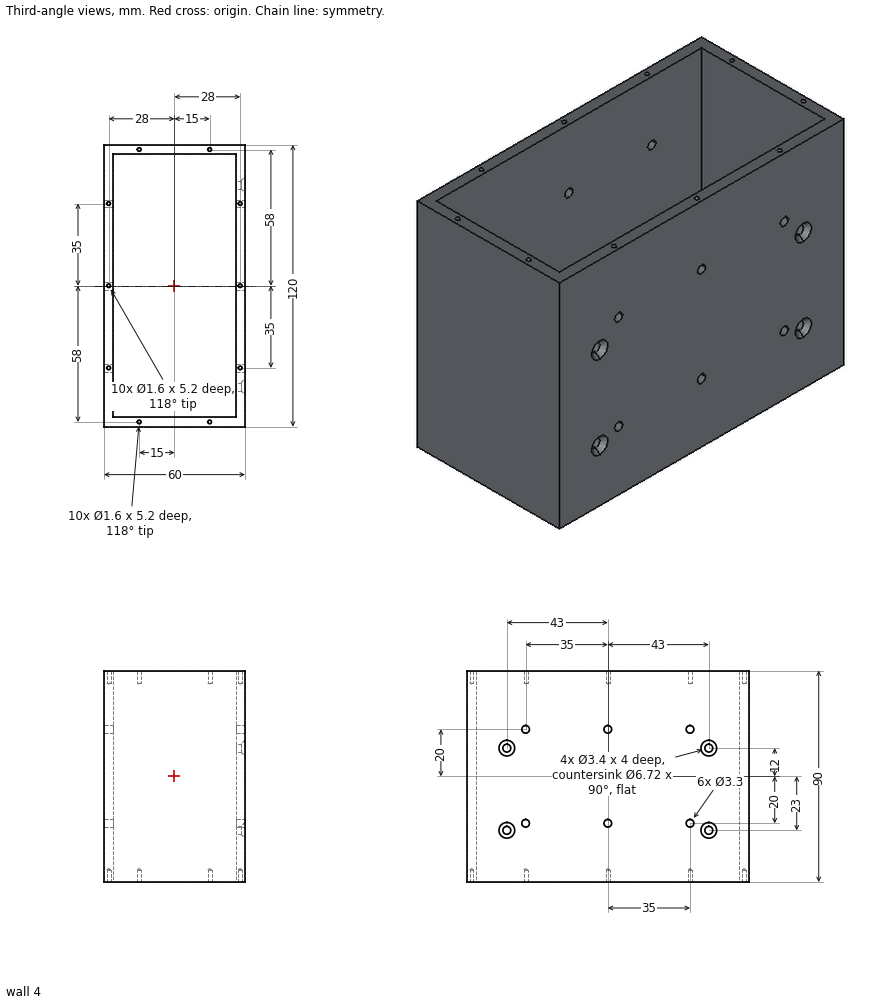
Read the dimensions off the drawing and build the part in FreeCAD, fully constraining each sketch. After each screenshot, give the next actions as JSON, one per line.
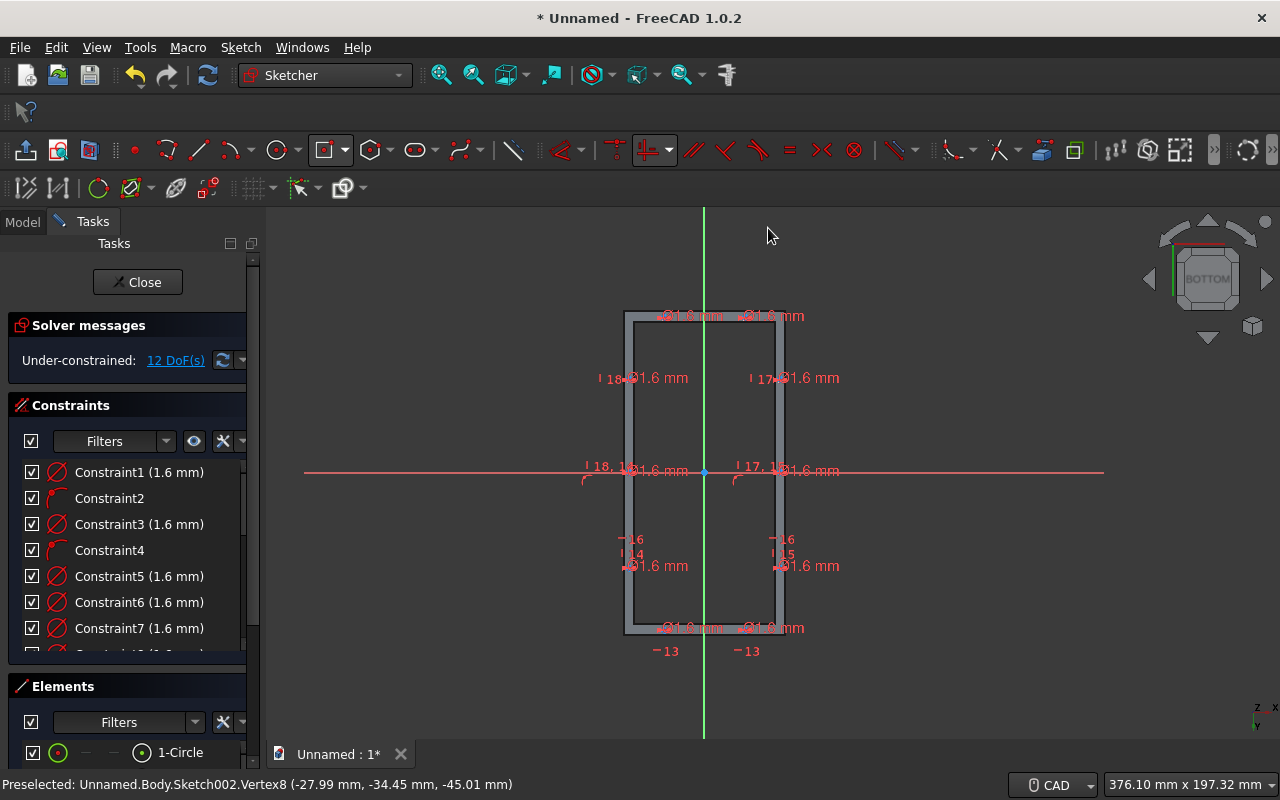
{"action": "left_click", "coordinate": [780, 380]}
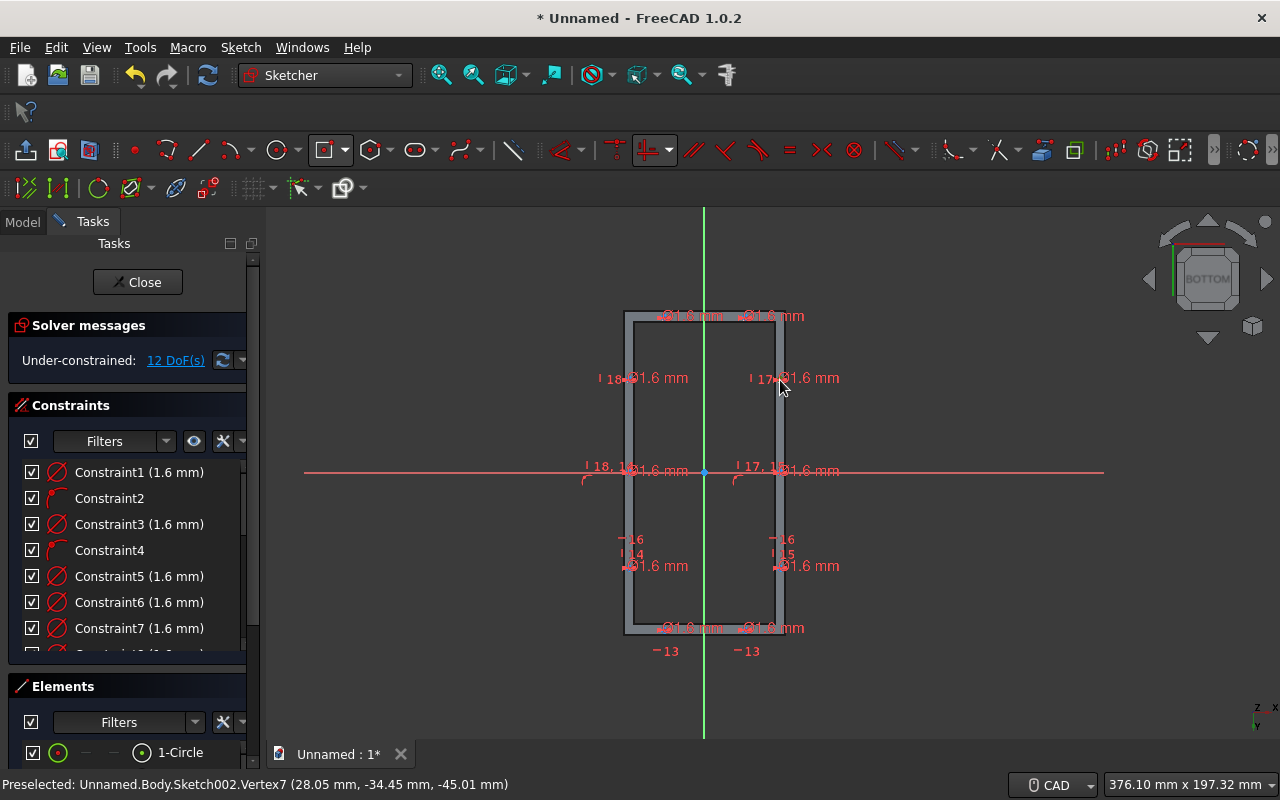
{"action": "left_click", "coordinate": [629, 380]}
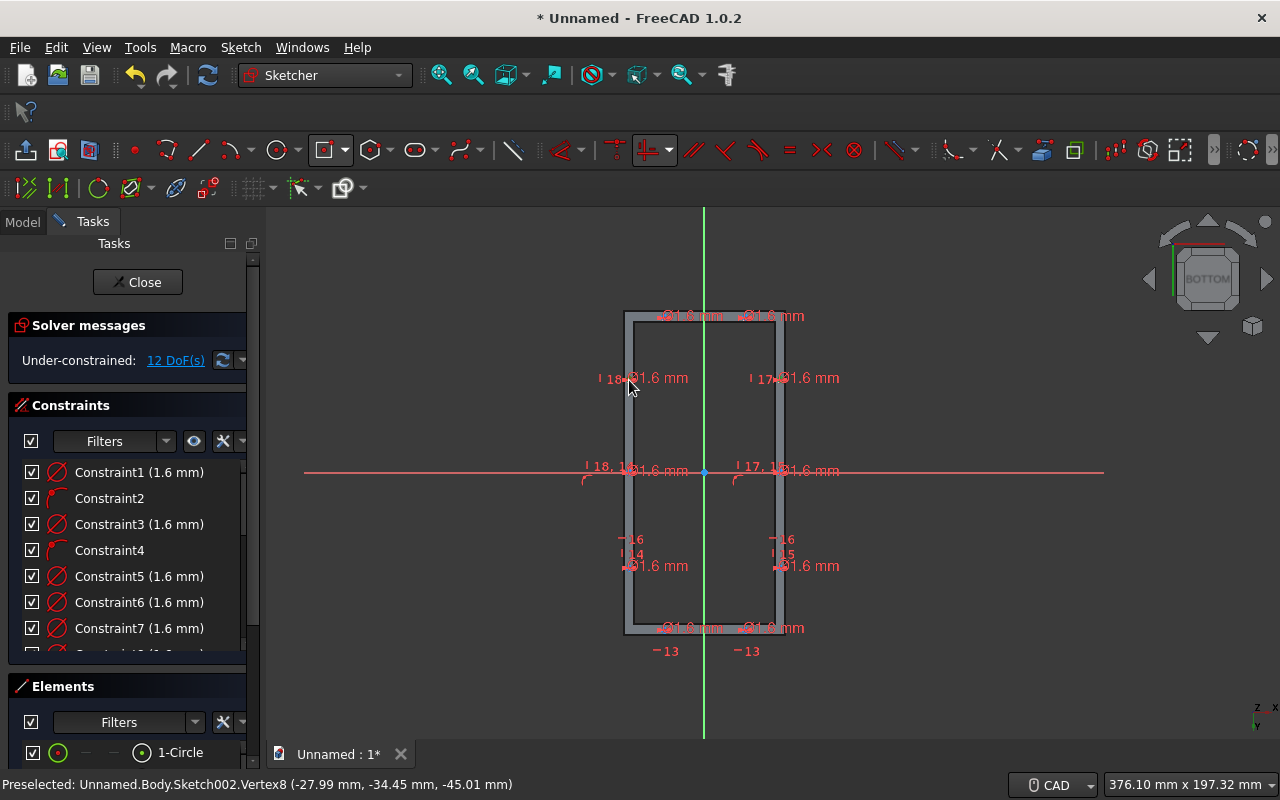
{"action": "key", "text": "h"}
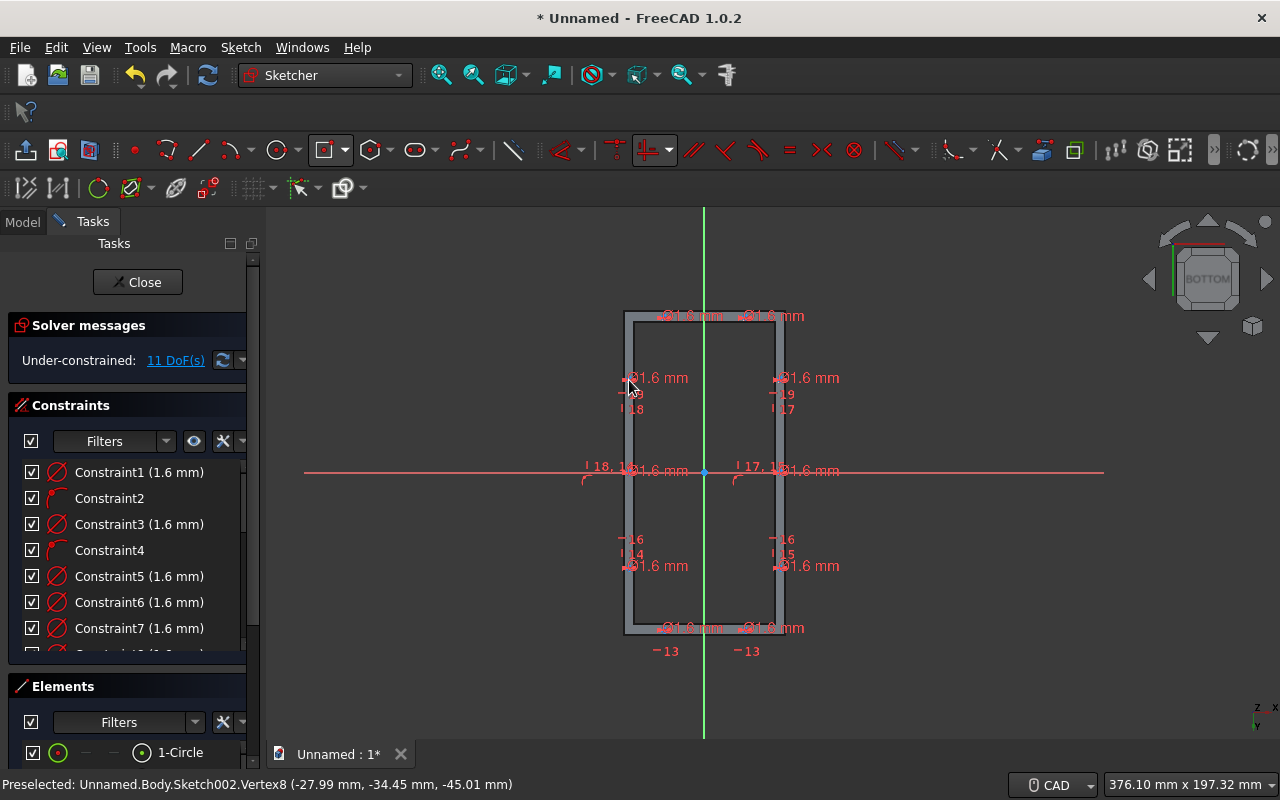
{"action": "left_click", "coordinate": [745, 318]}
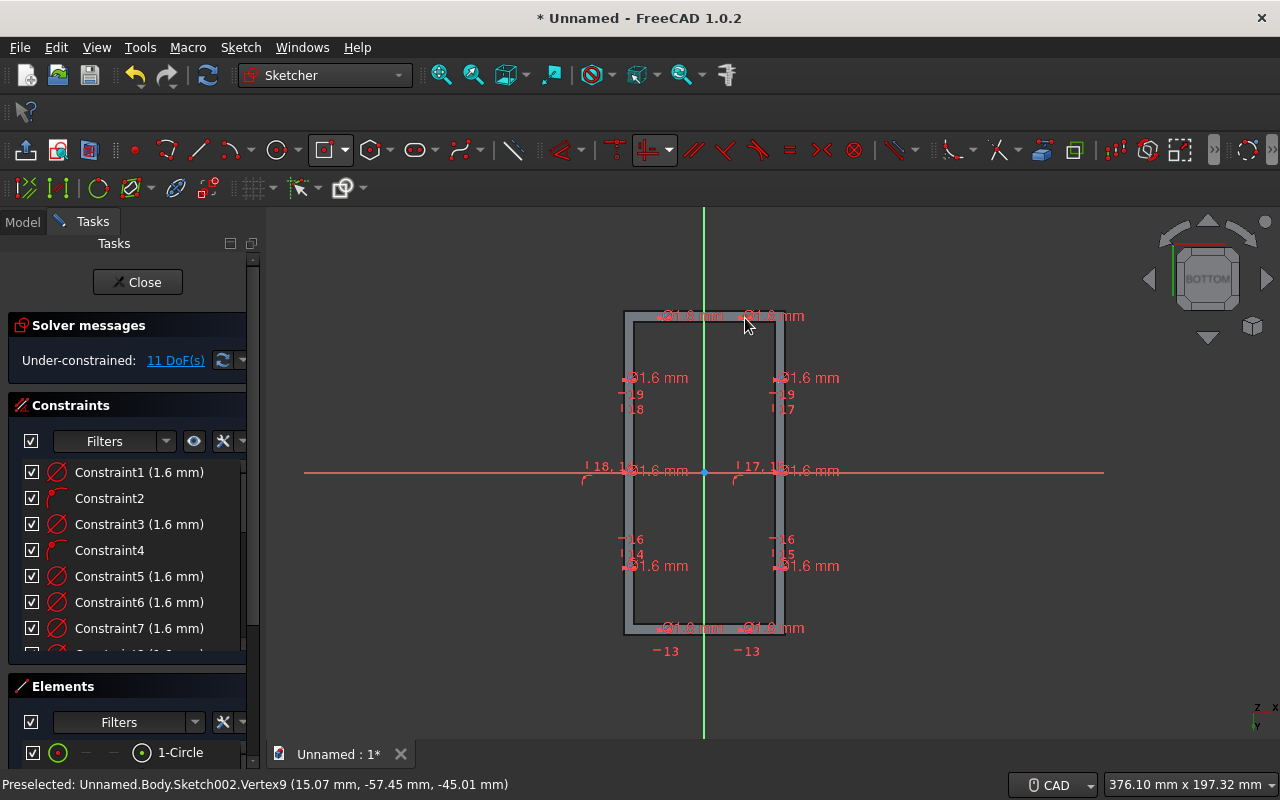
{"action": "left_click", "coordinate": [664, 318]}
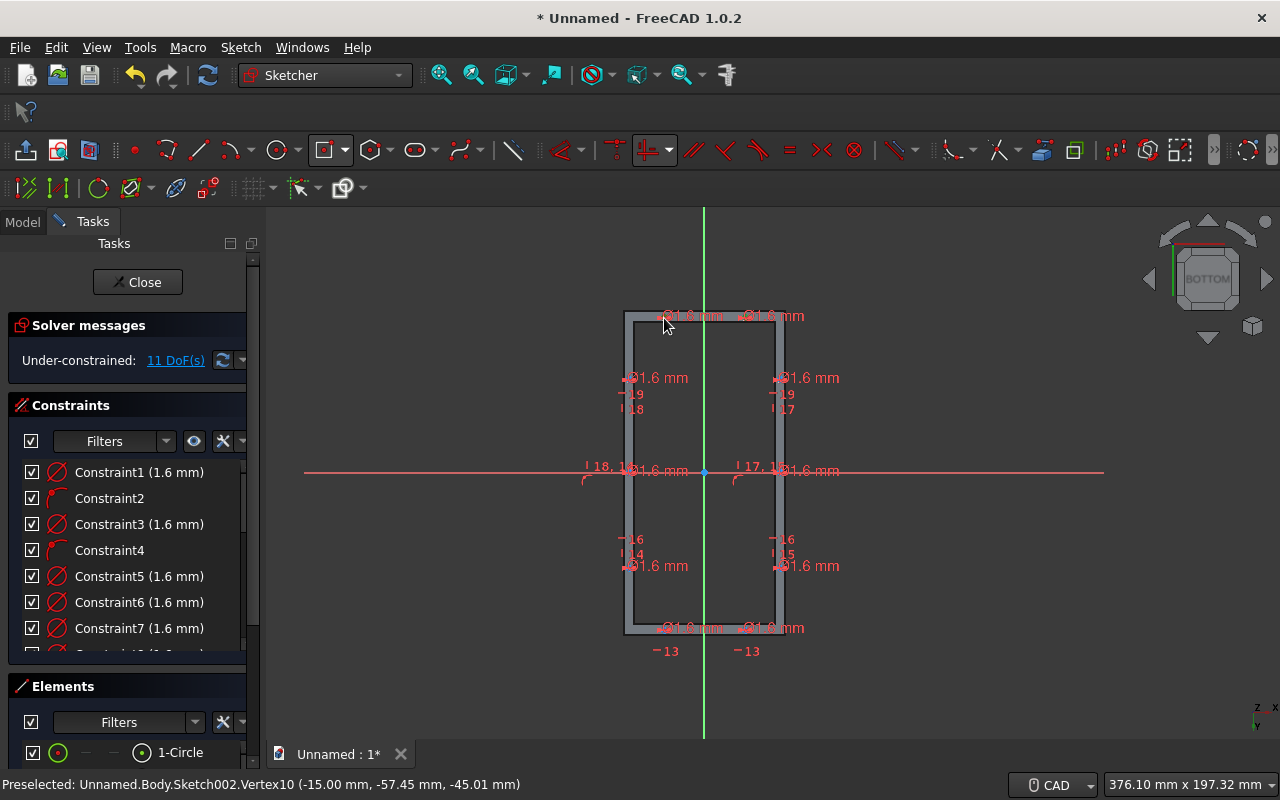
{"action": "left_click", "coordinate": [672, 150]}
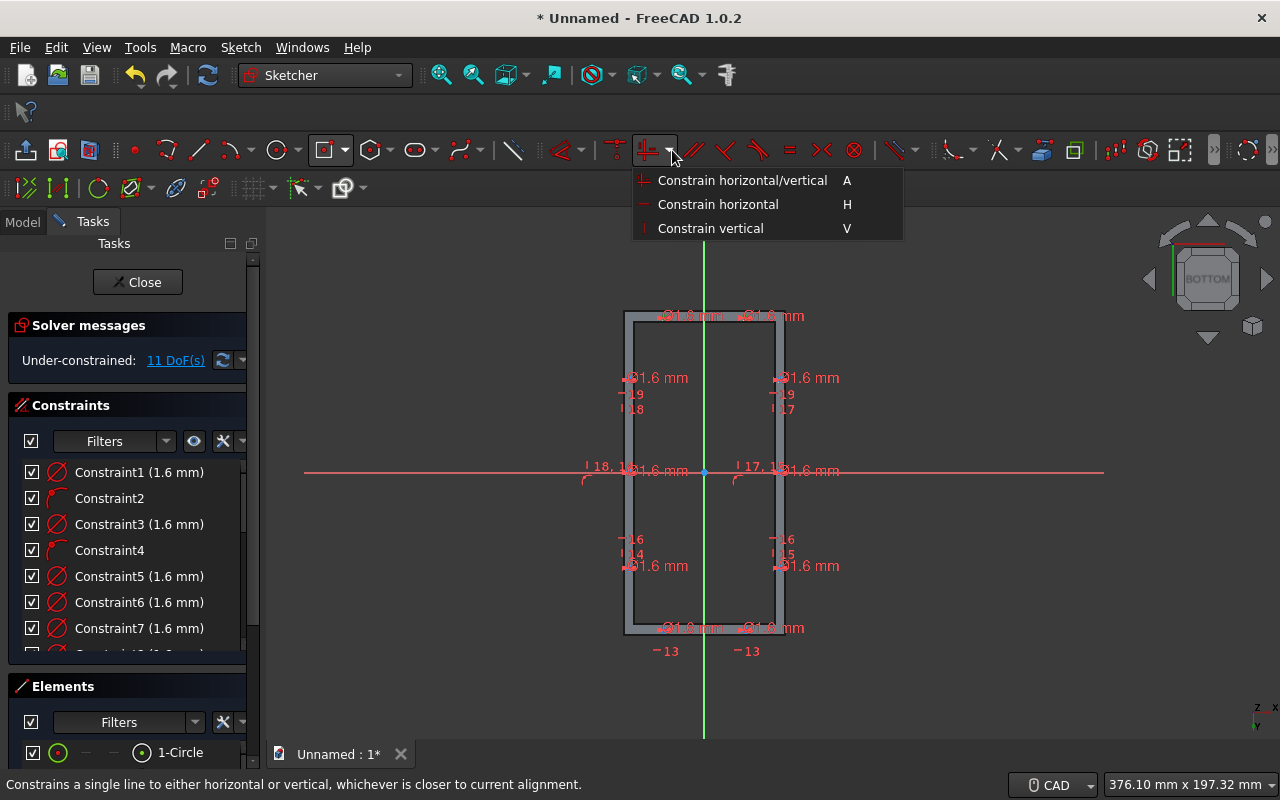
{"action": "left_click", "coordinate": [768, 204]}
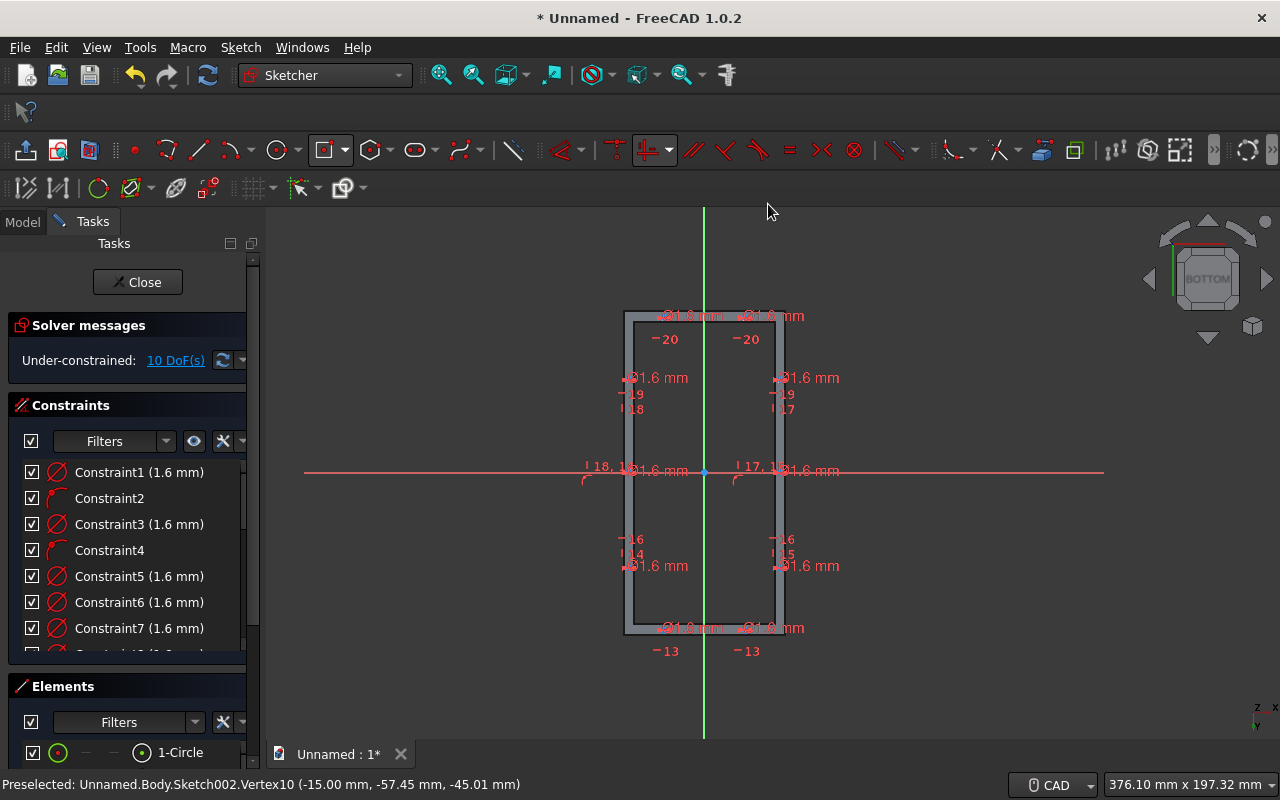
{"action": "left_click", "coordinate": [745, 630]}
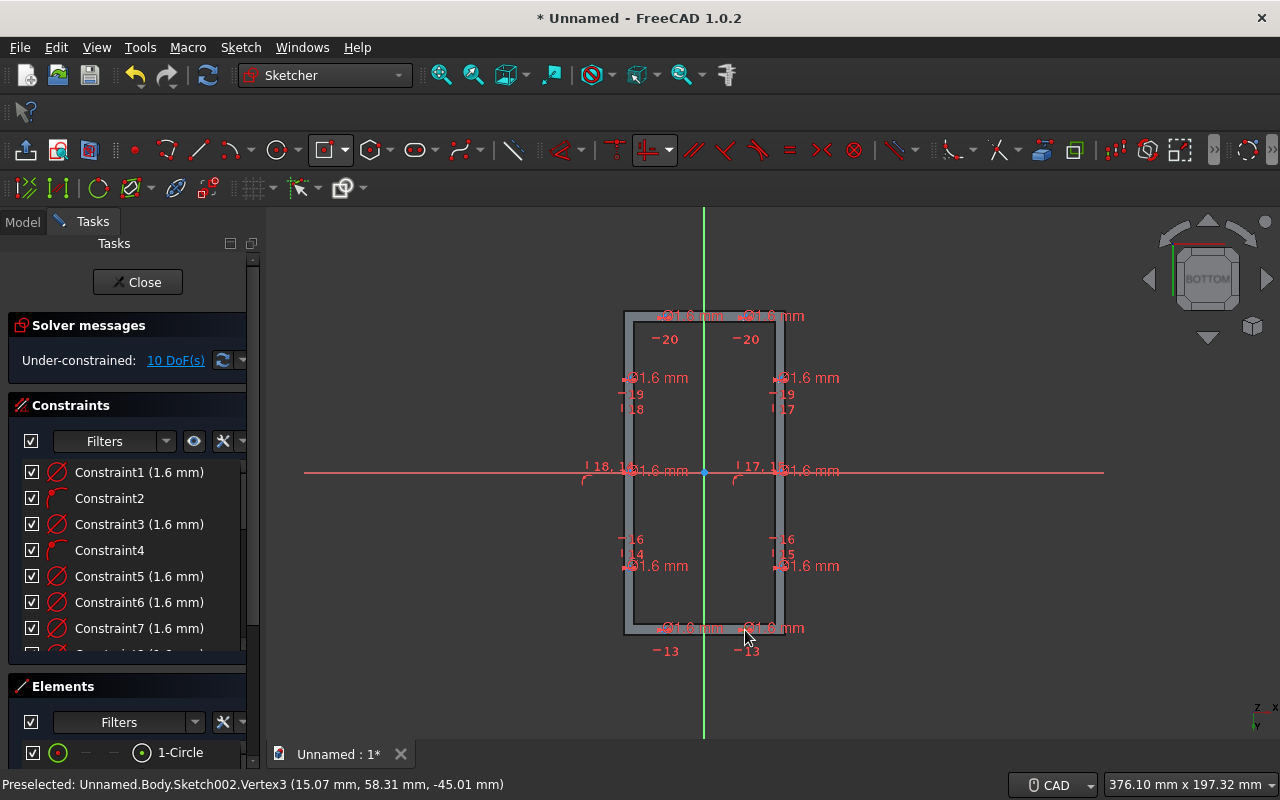
{"action": "left_click", "coordinate": [745, 318]}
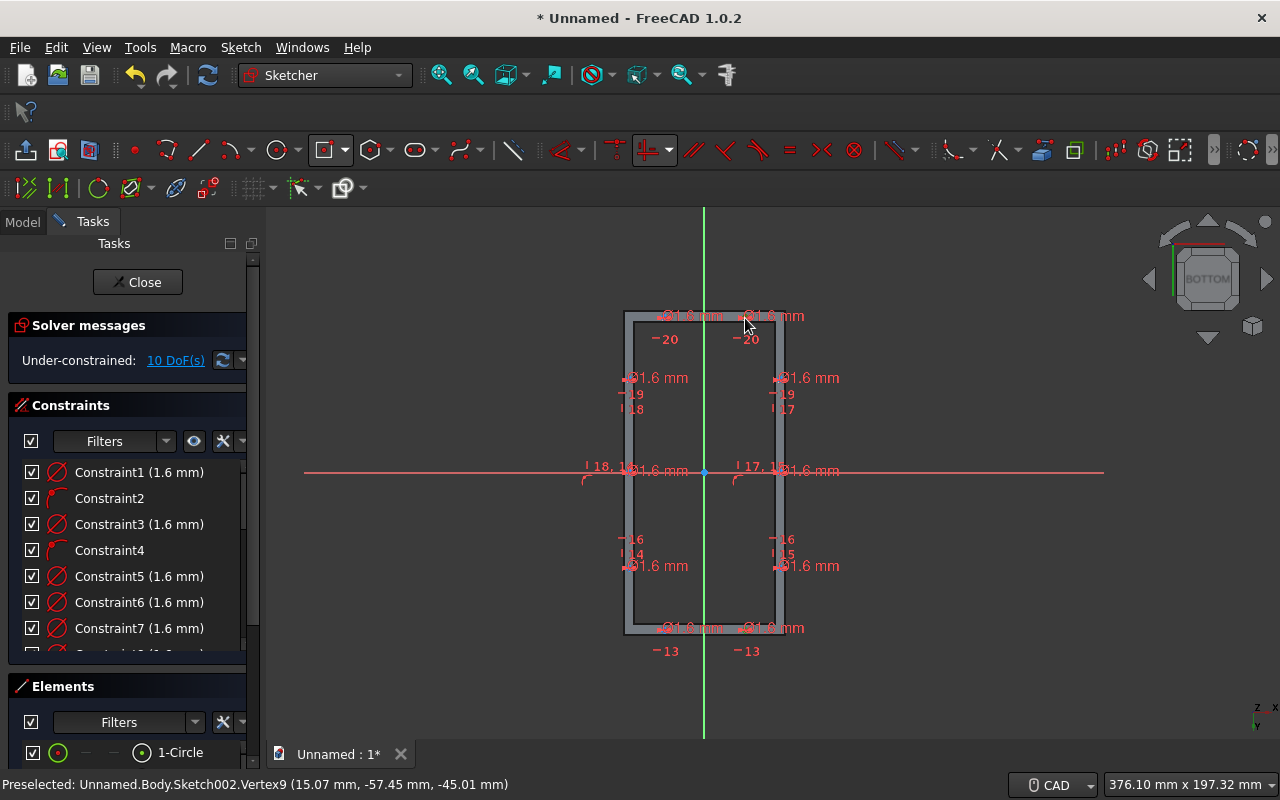
{"action": "left_click", "coordinate": [353, 473]}